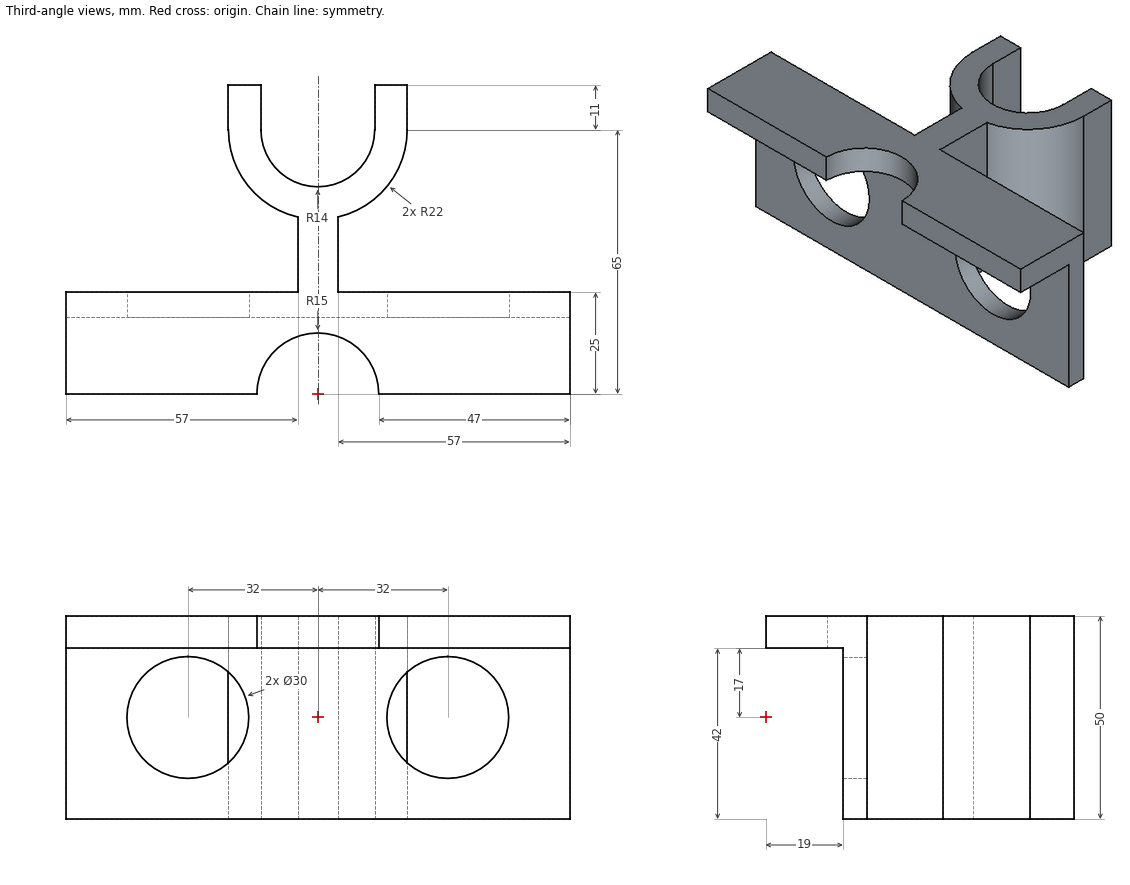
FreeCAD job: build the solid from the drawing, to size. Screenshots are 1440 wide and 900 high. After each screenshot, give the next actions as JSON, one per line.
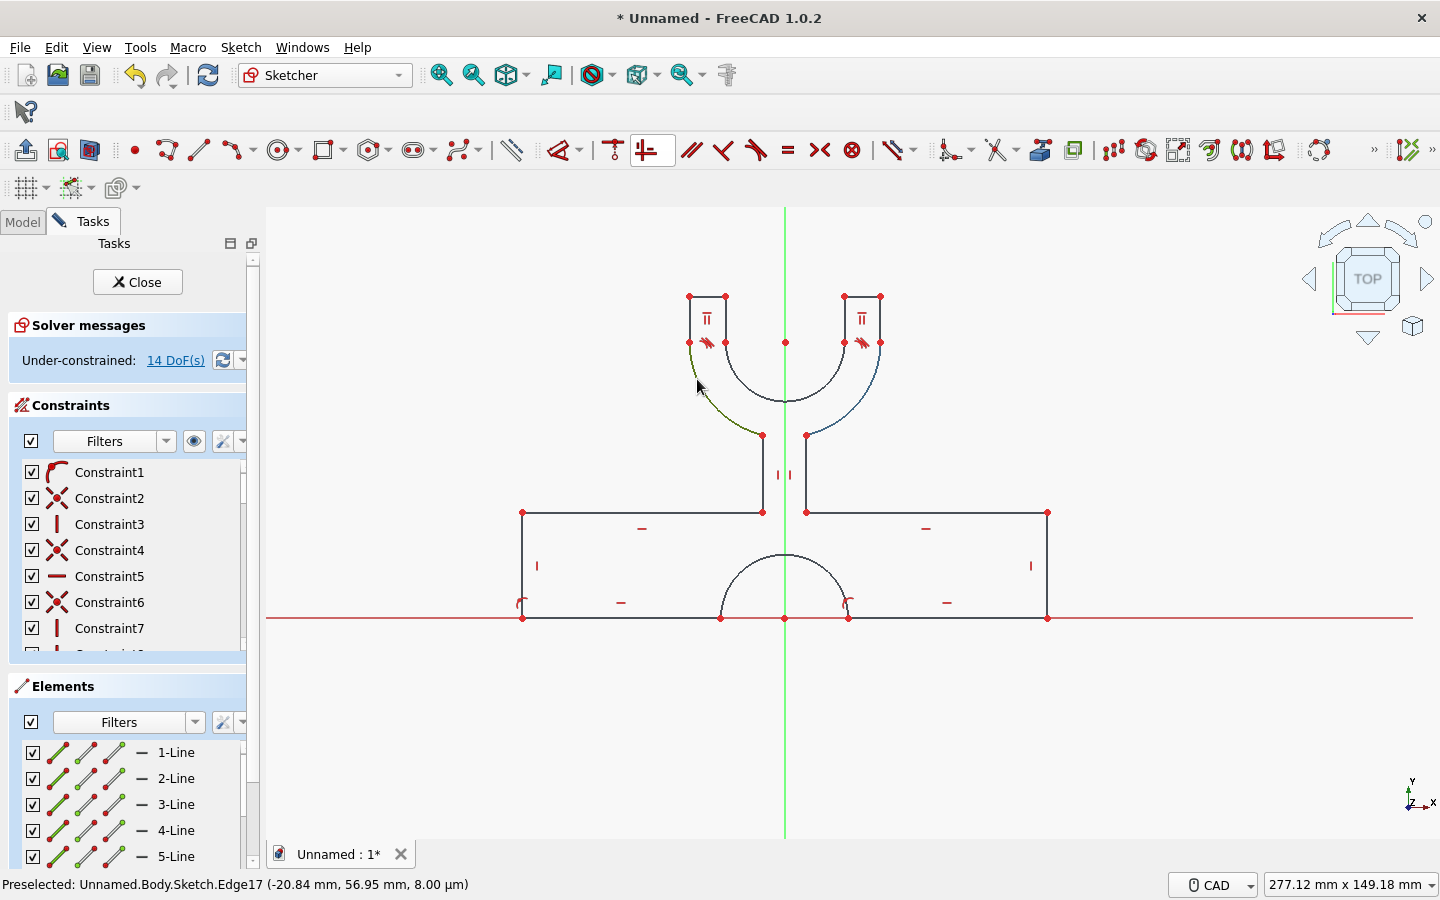
{"action": "left_click", "coordinate": [788, 150]}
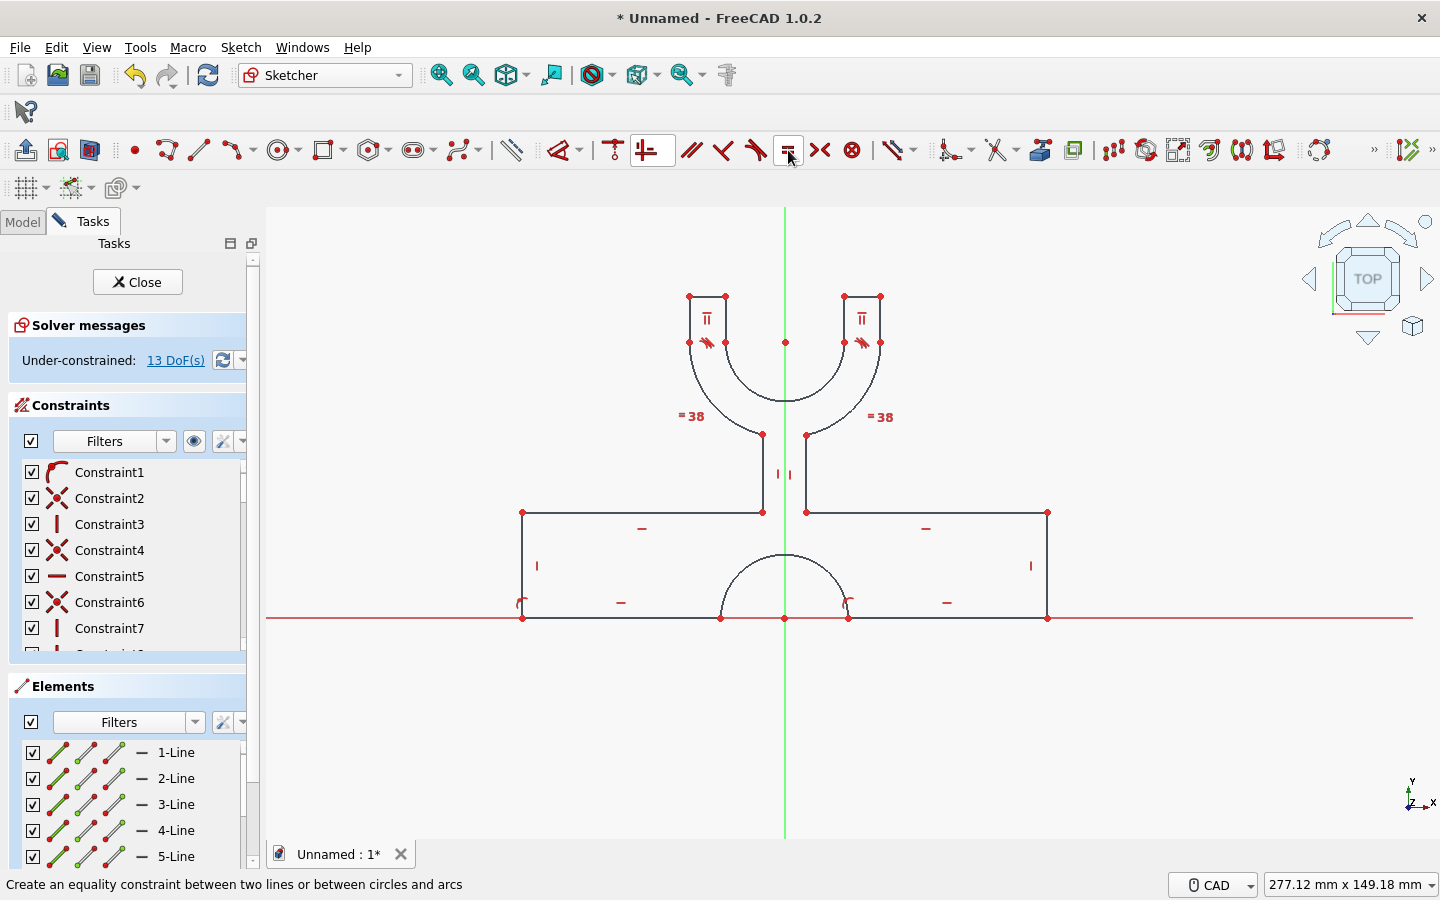
{"action": "left_click", "coordinate": [785, 342]}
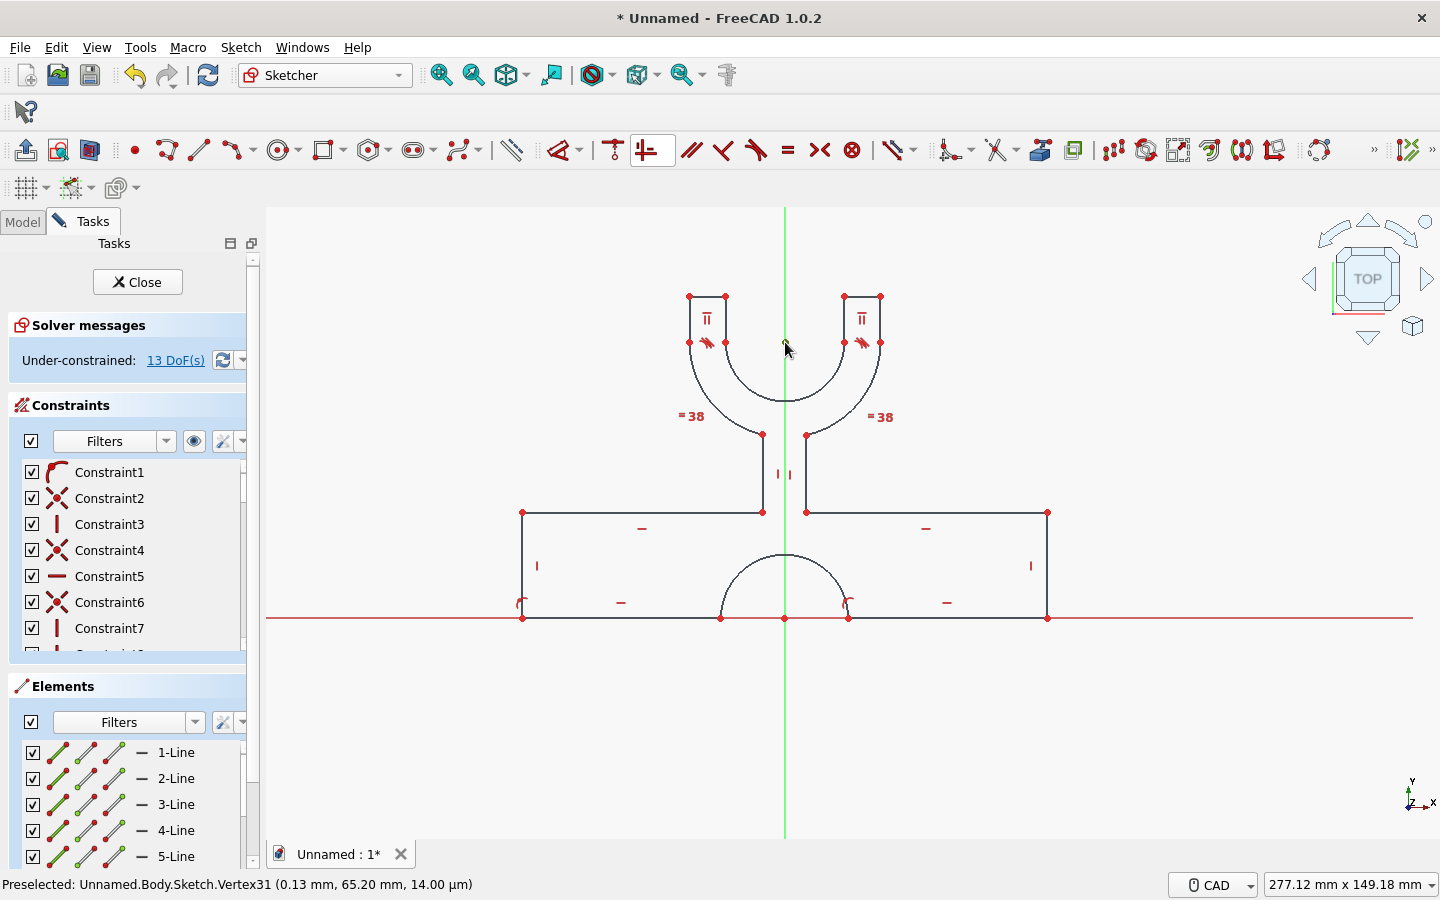
{"action": "left_click", "coordinate": [785, 770]}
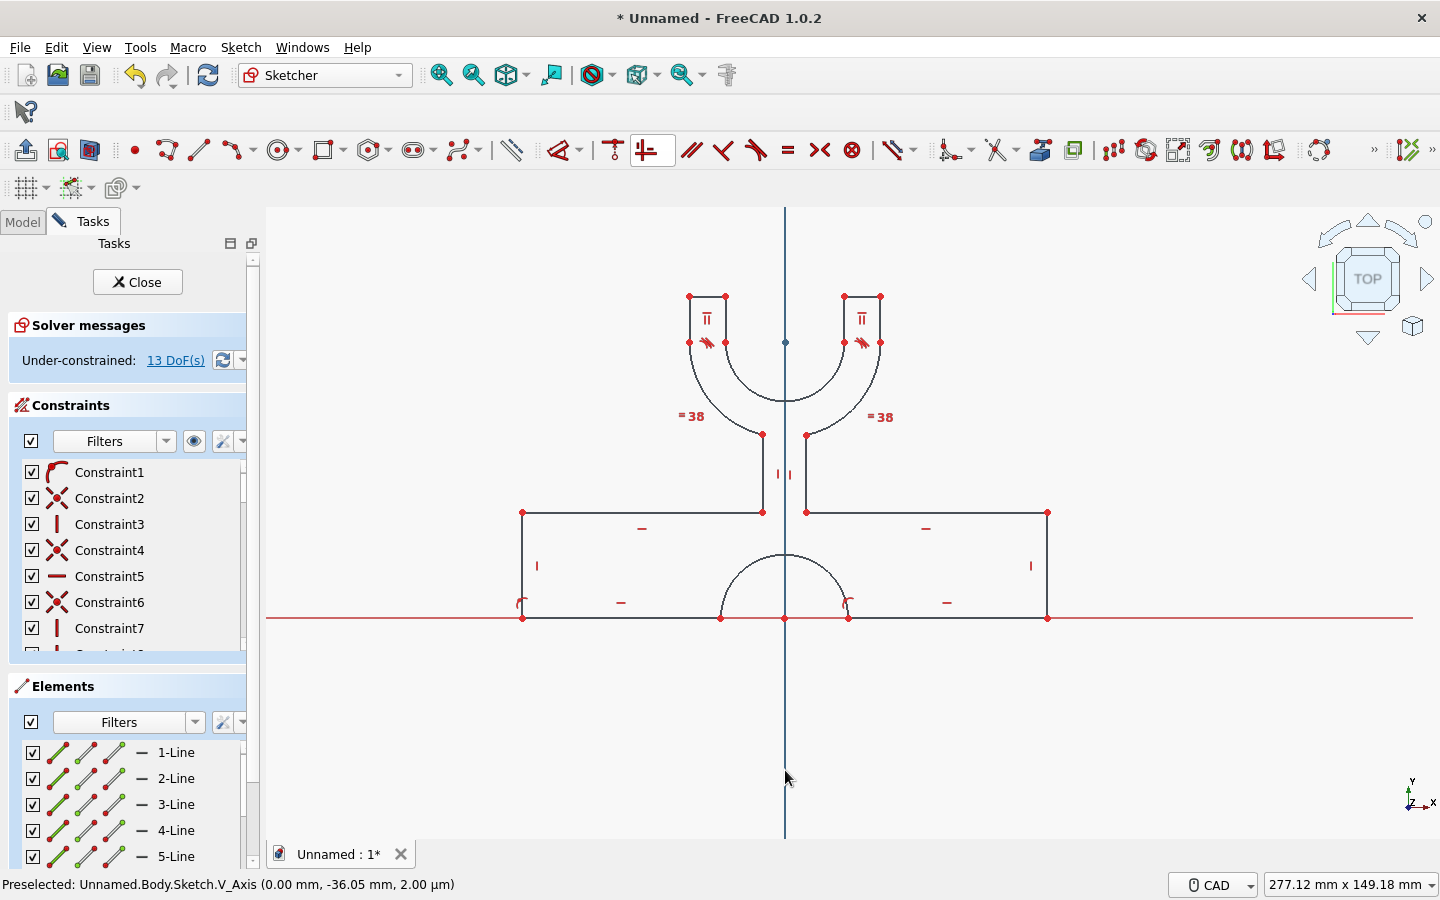
{"action": "left_click", "coordinate": [614, 150]}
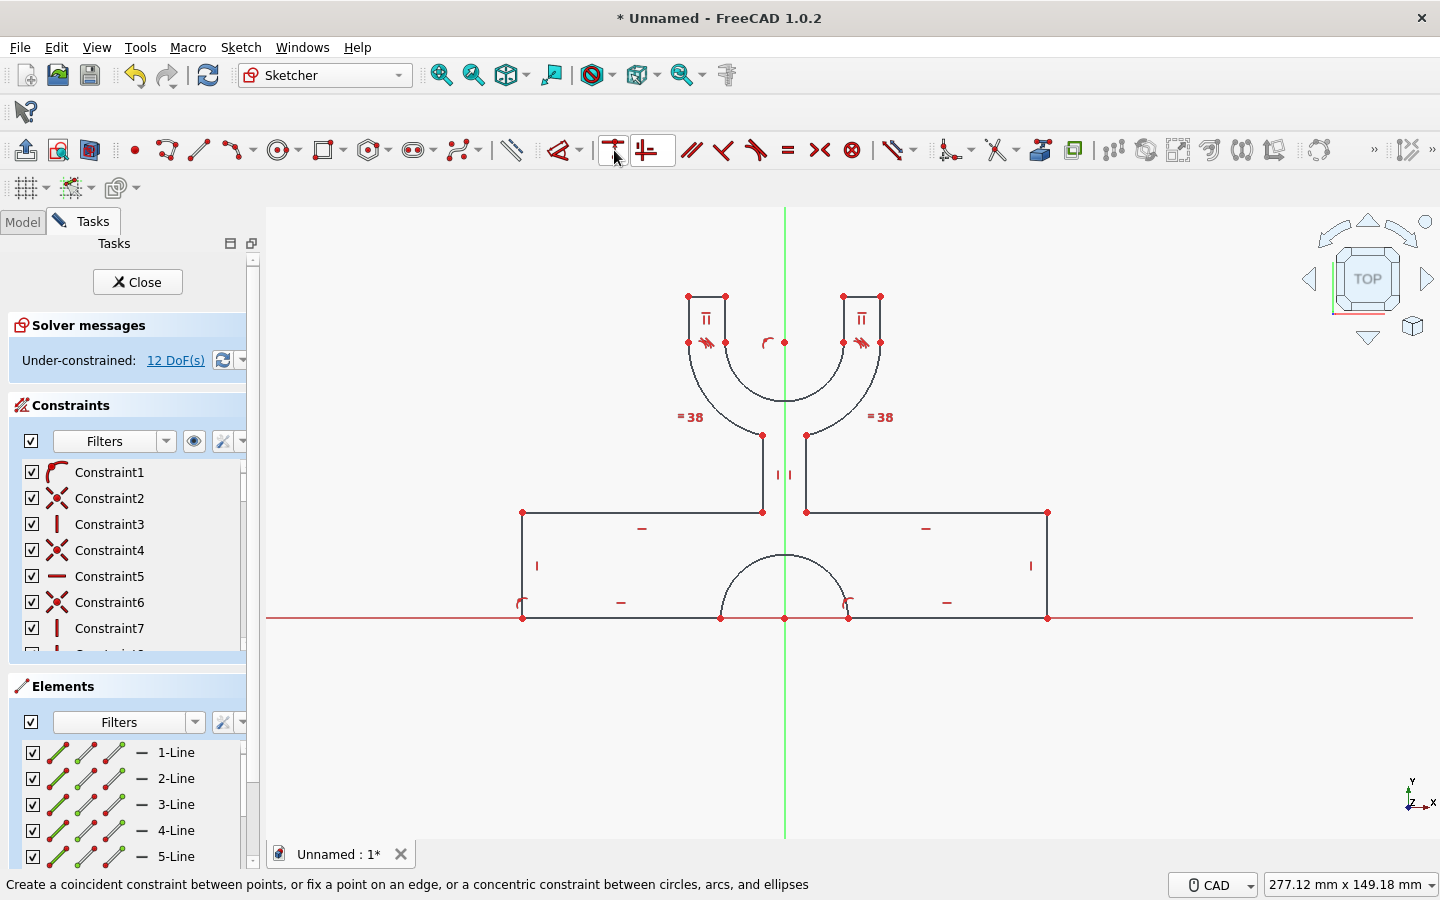
{"action": "left_click", "coordinate": [806, 513]}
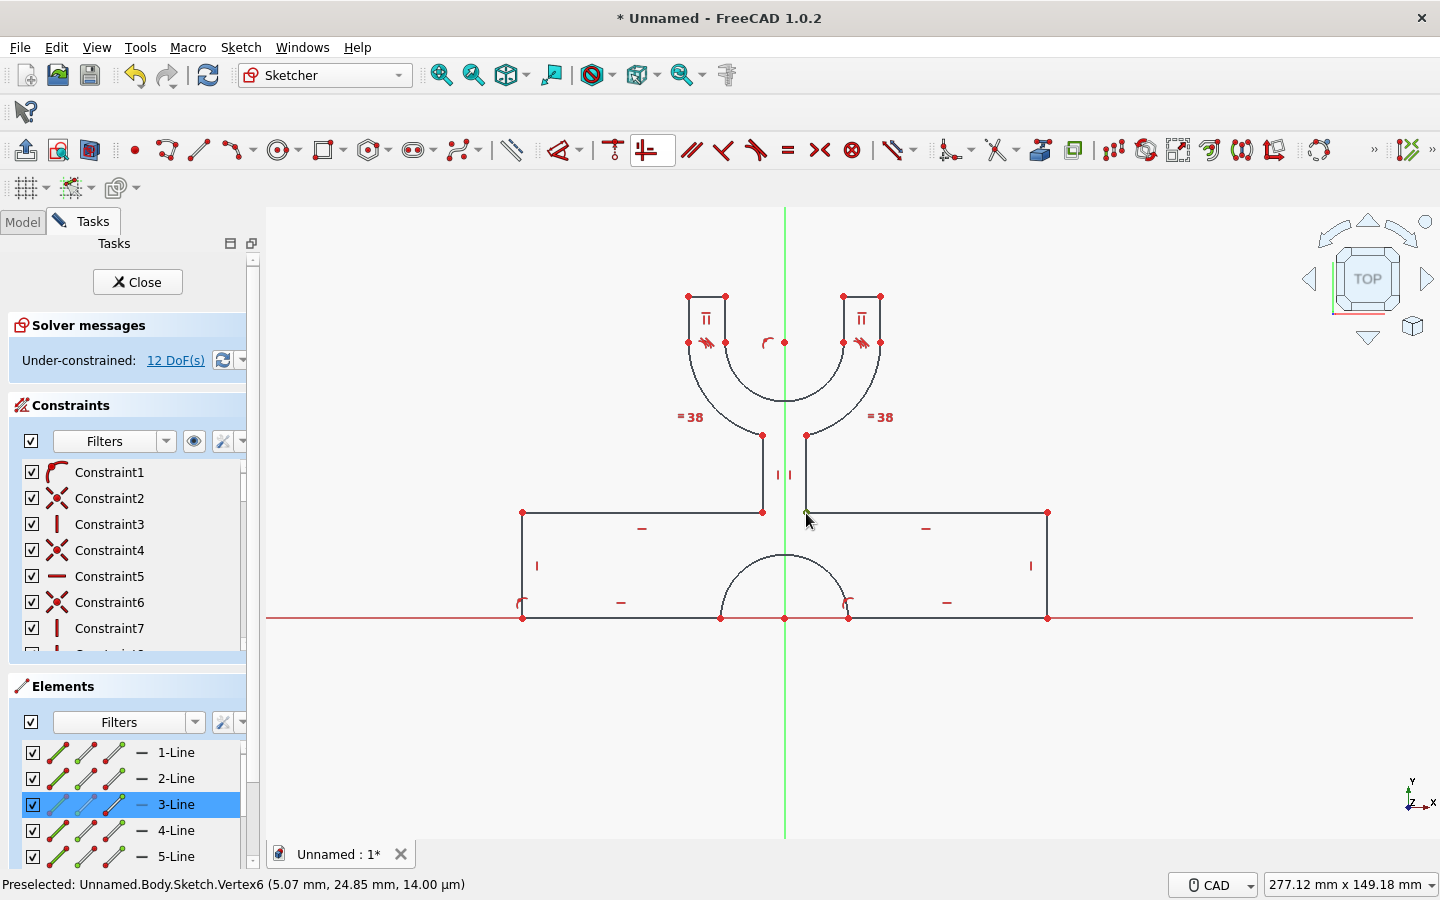
{"action": "left_click", "coordinate": [763, 513]}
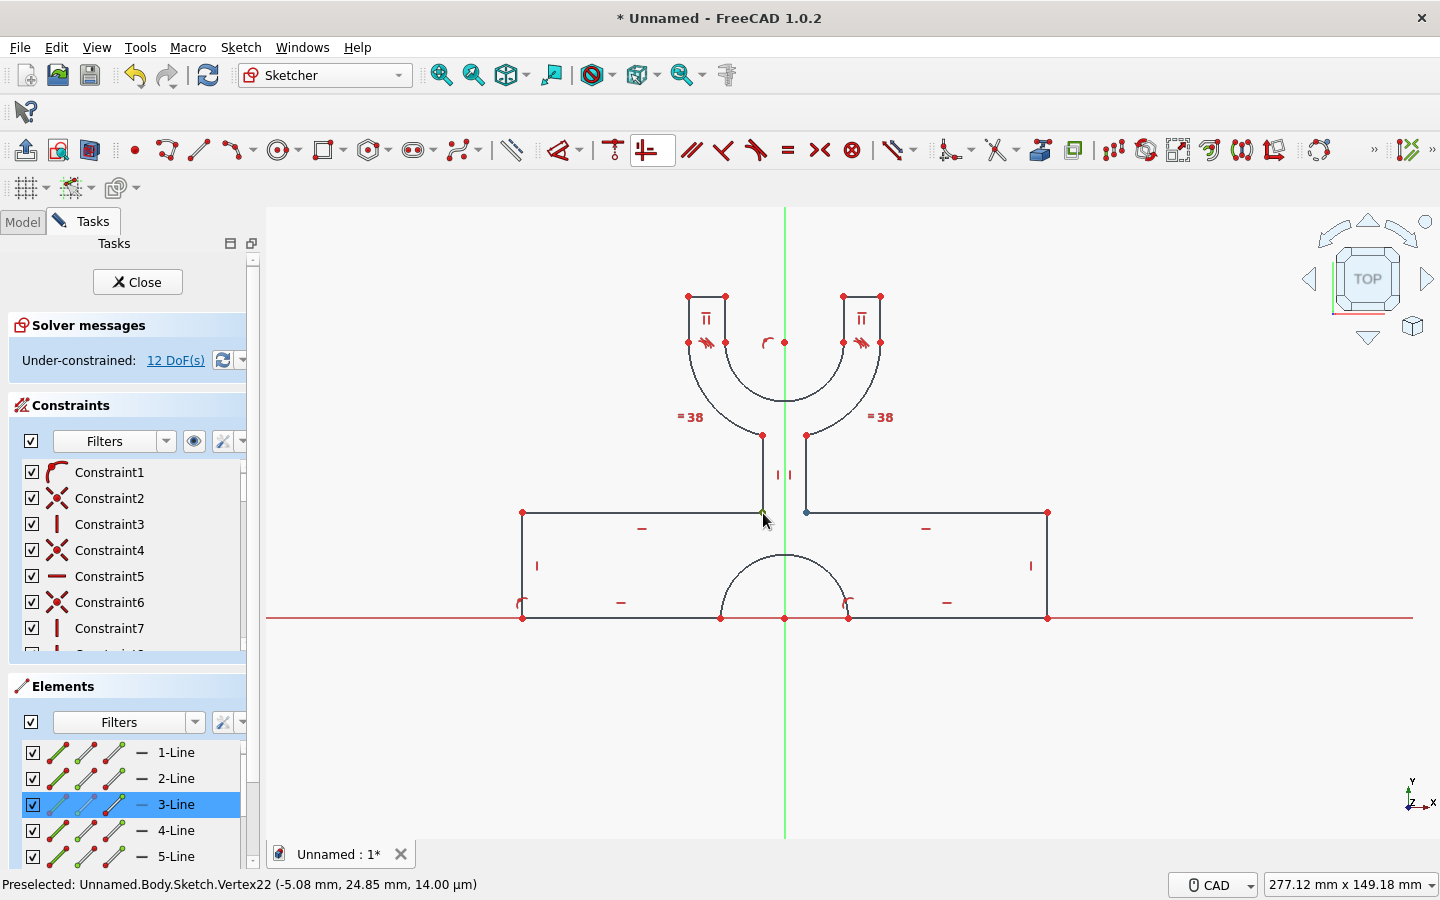
{"action": "left_click", "coordinate": [785, 770]}